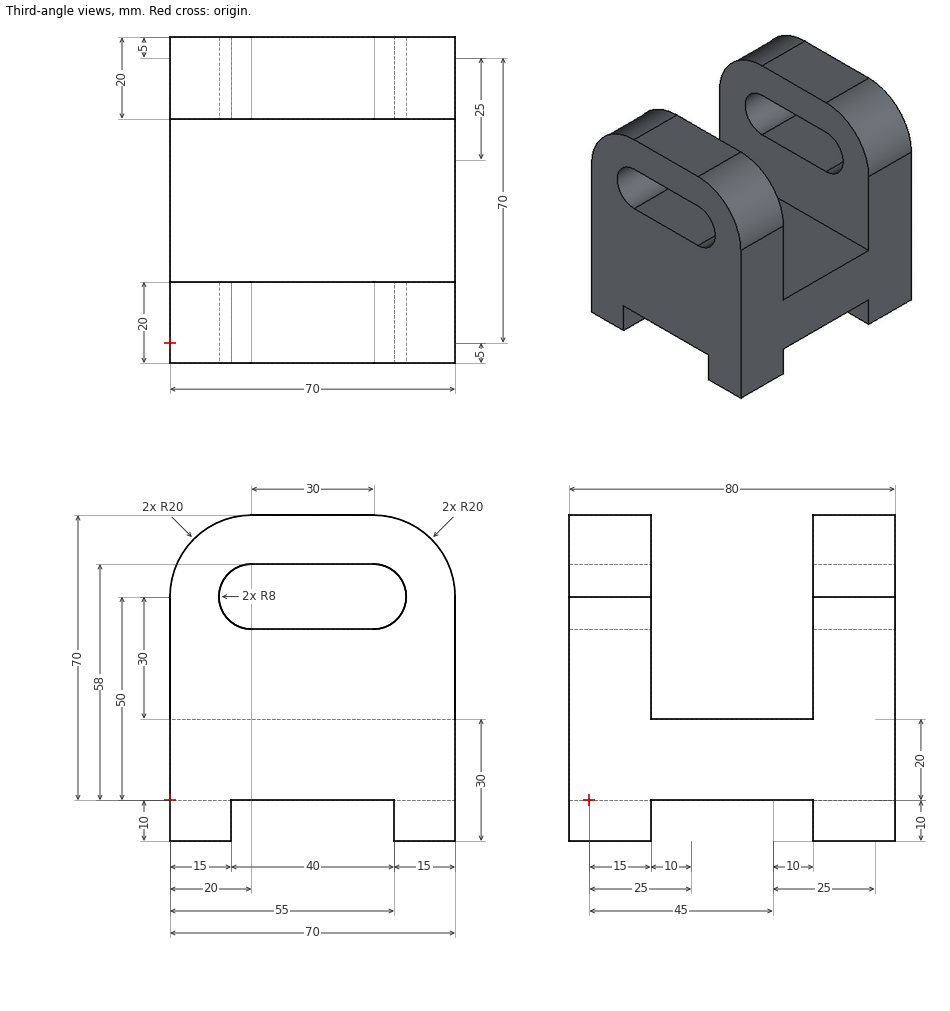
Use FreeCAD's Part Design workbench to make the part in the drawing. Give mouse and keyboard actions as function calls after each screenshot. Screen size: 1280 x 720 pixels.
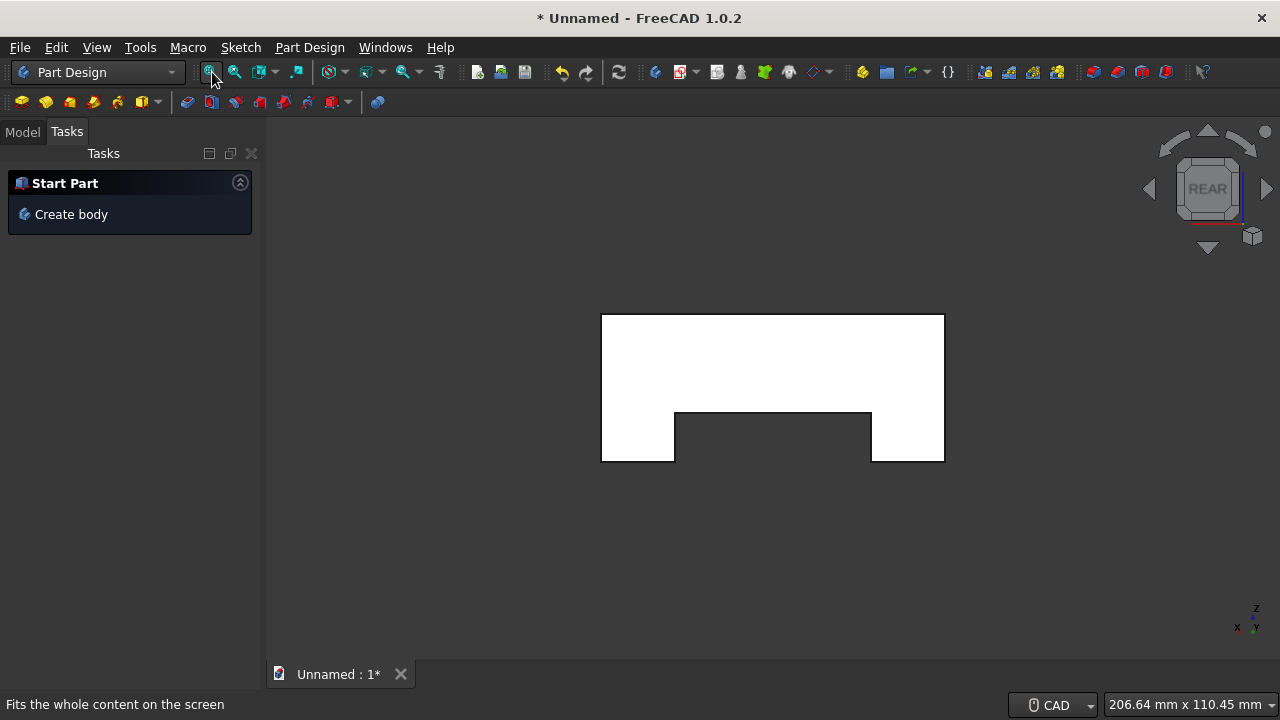
key(0)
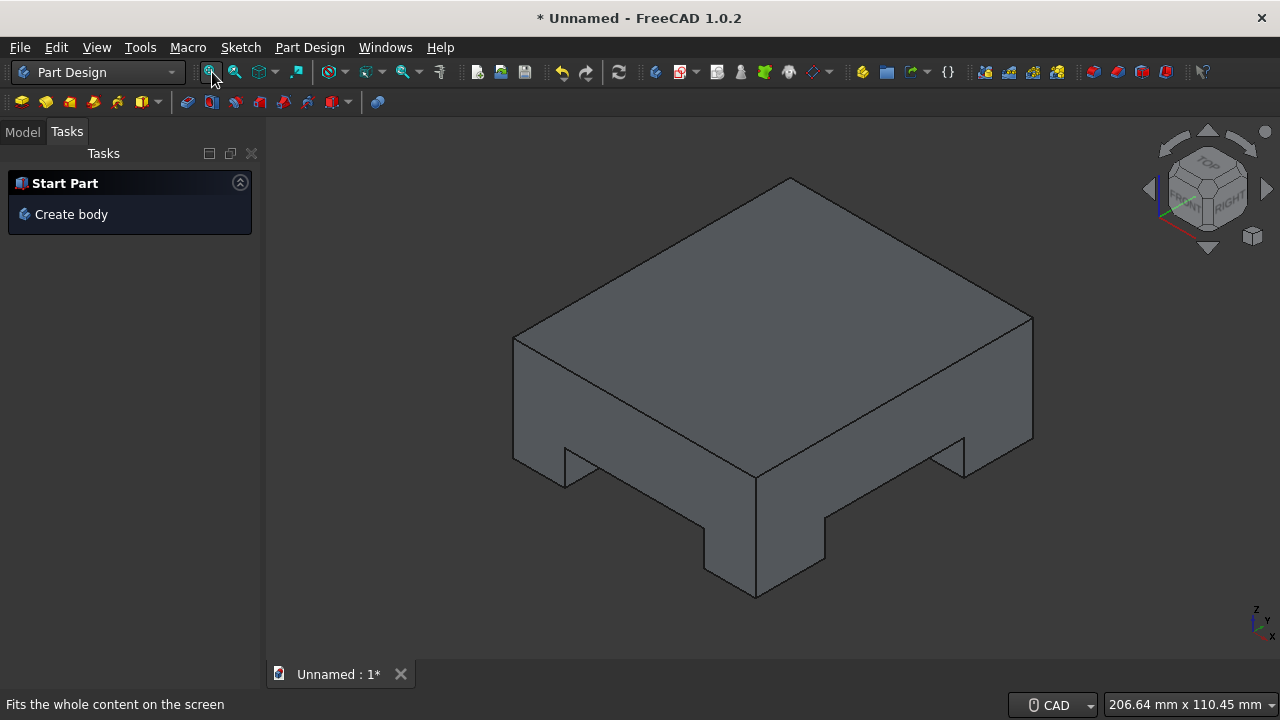
click(704, 490)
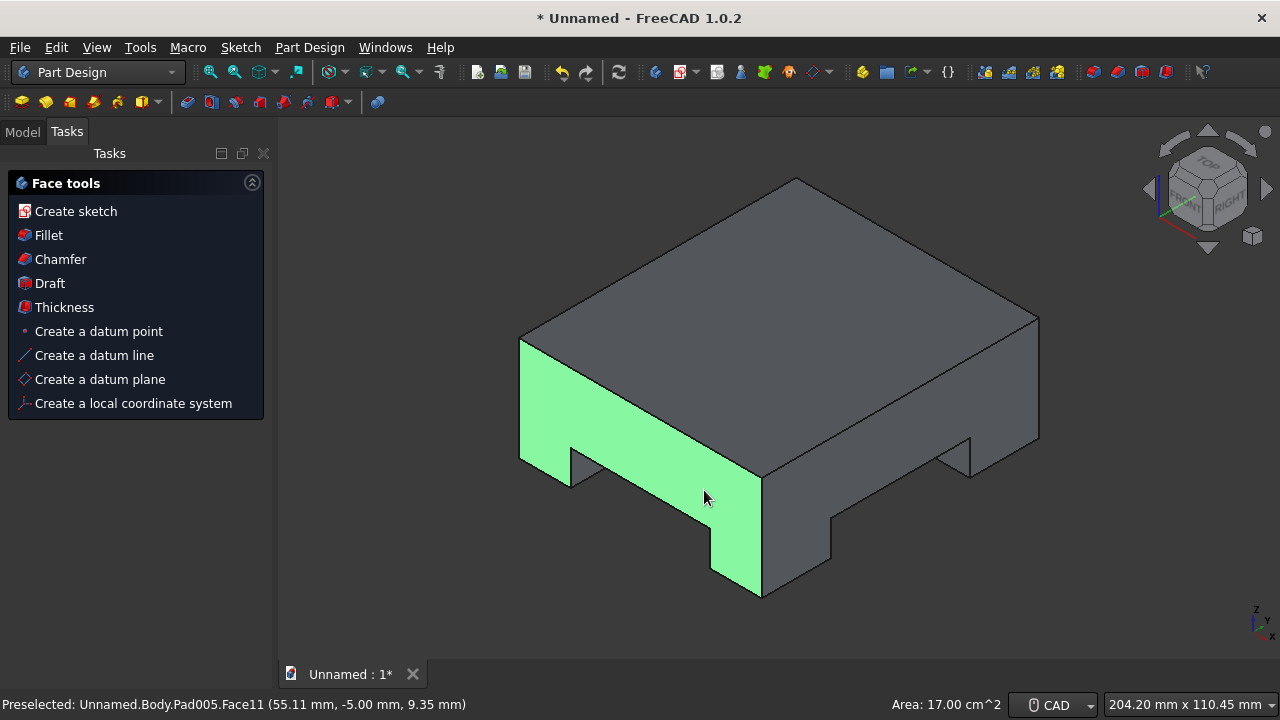
click(680, 72)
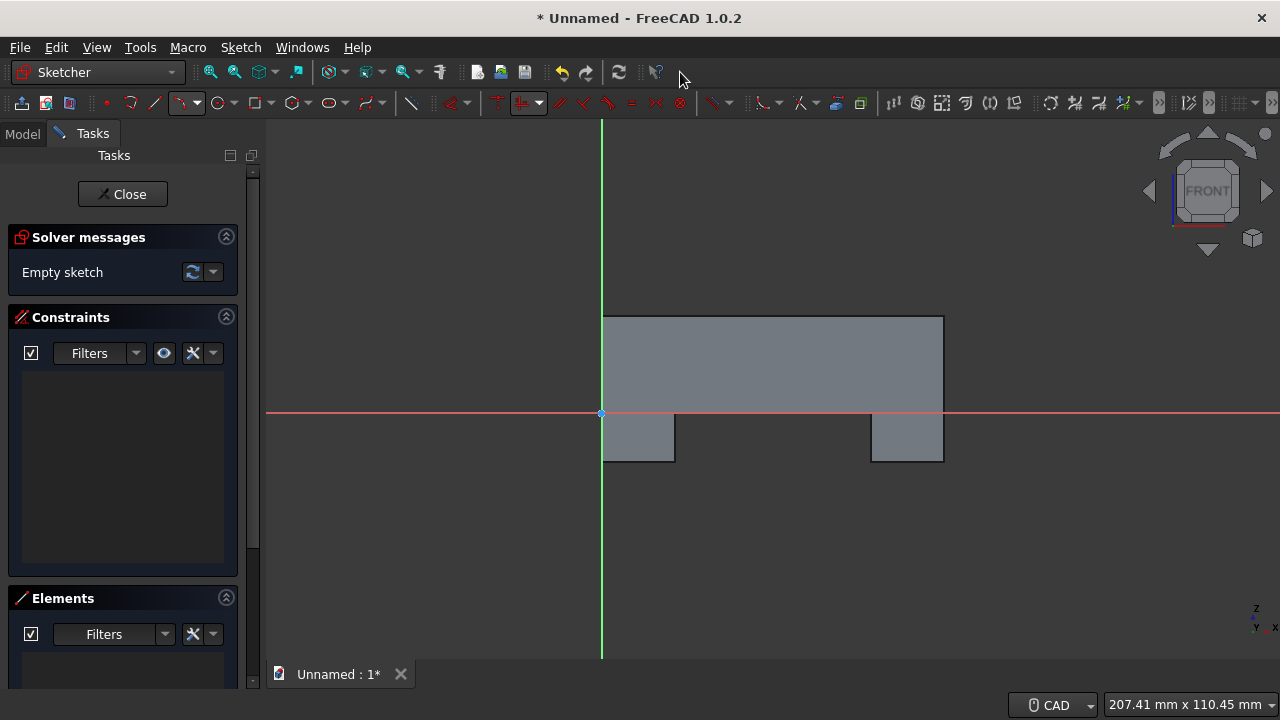
scroll(395, 631, down, 1)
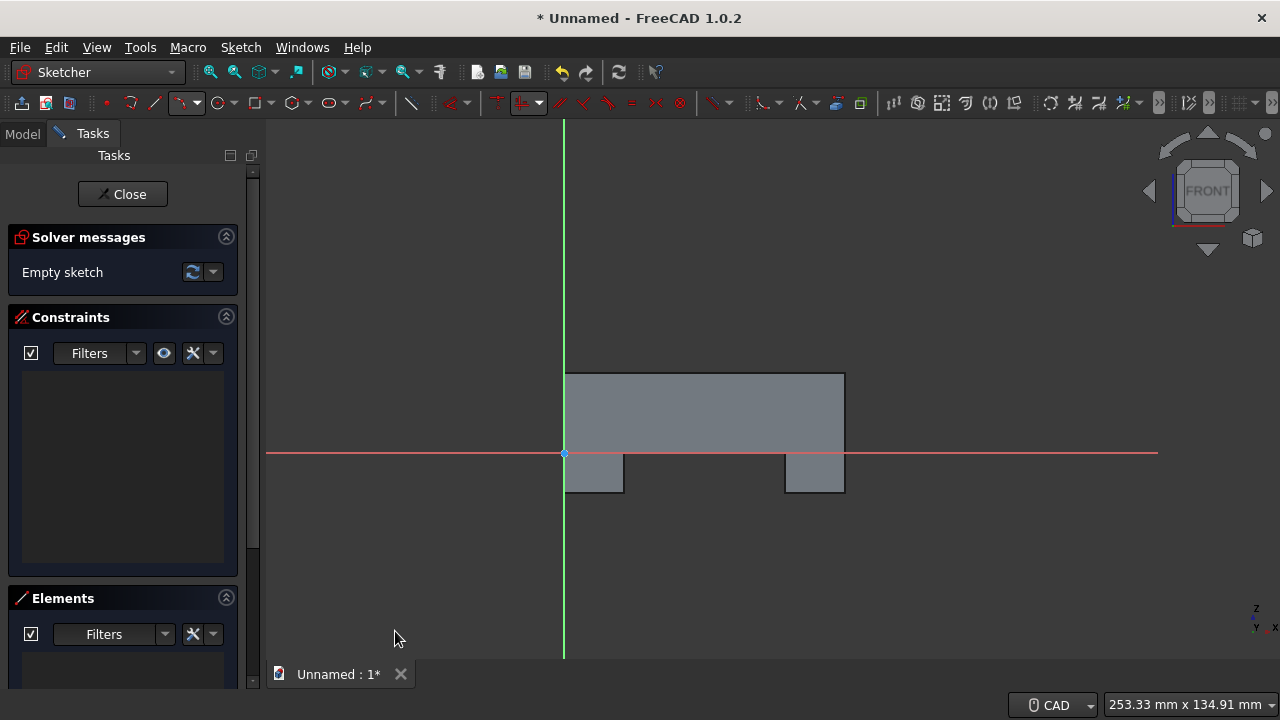
key(g)
key(m)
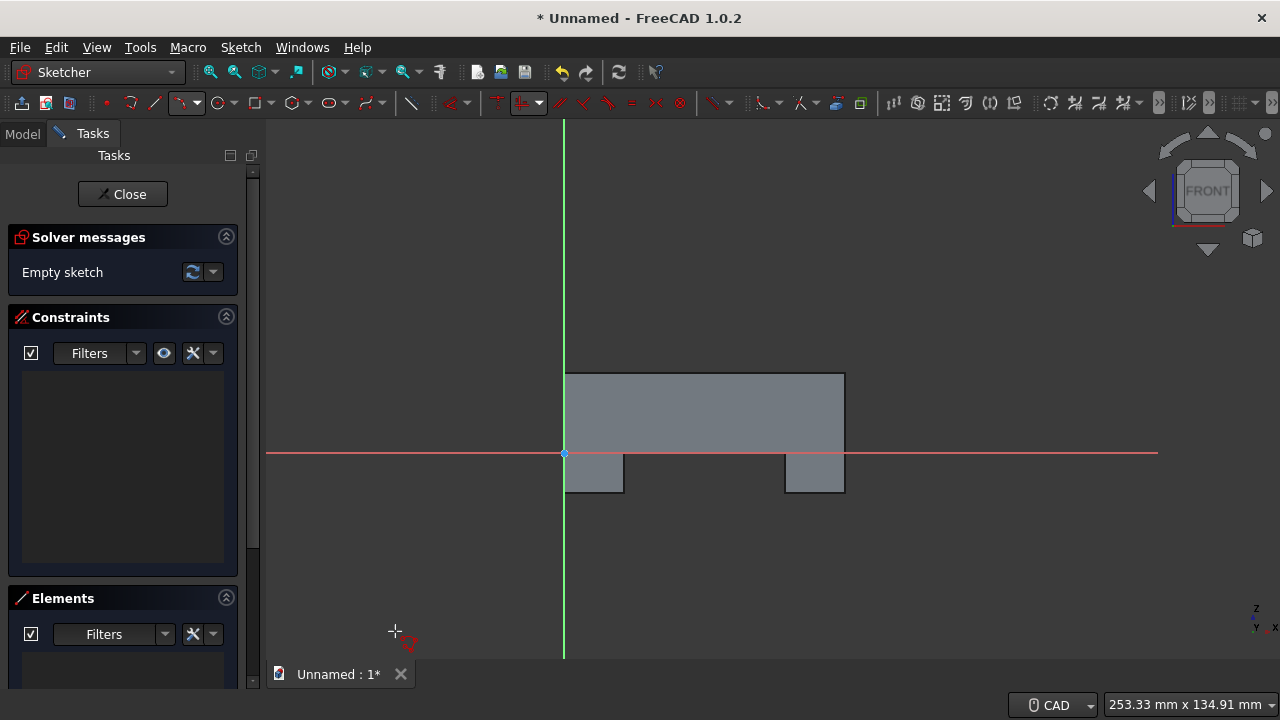
click(564, 253)
click(573, 373)
click(845, 373)
click(845, 253)
right_click(845, 253)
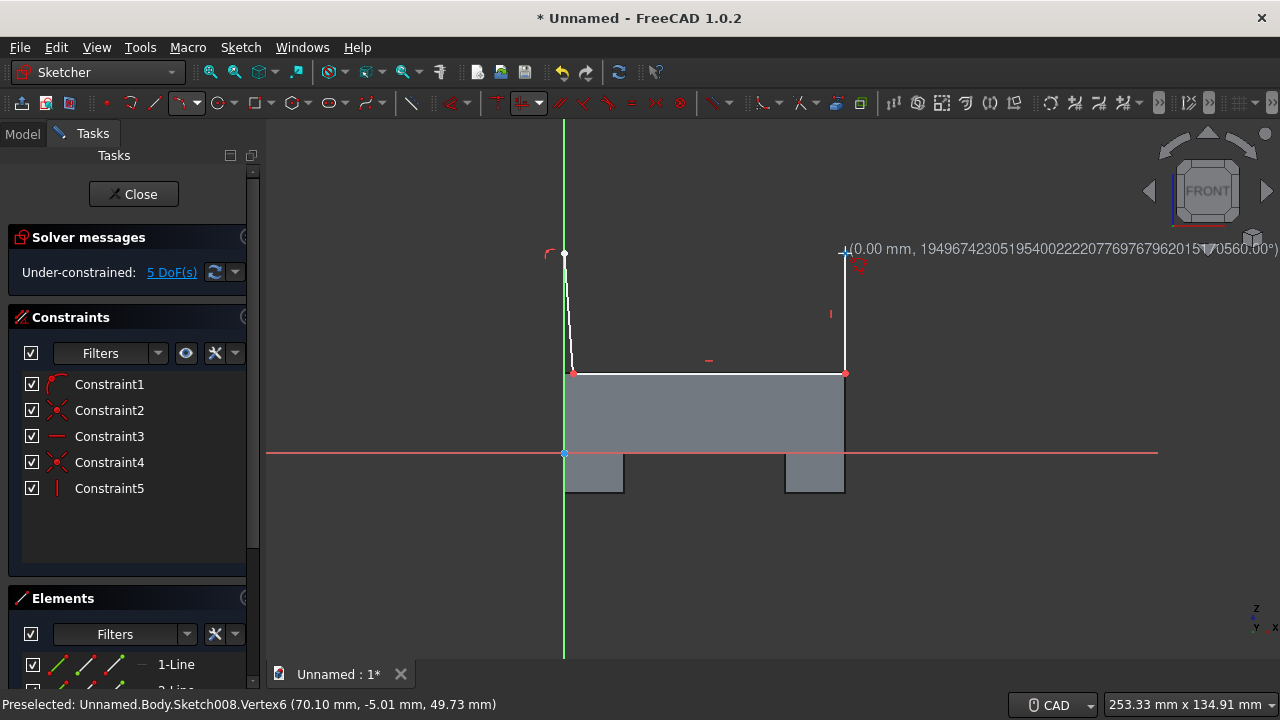
key(g)
key(l)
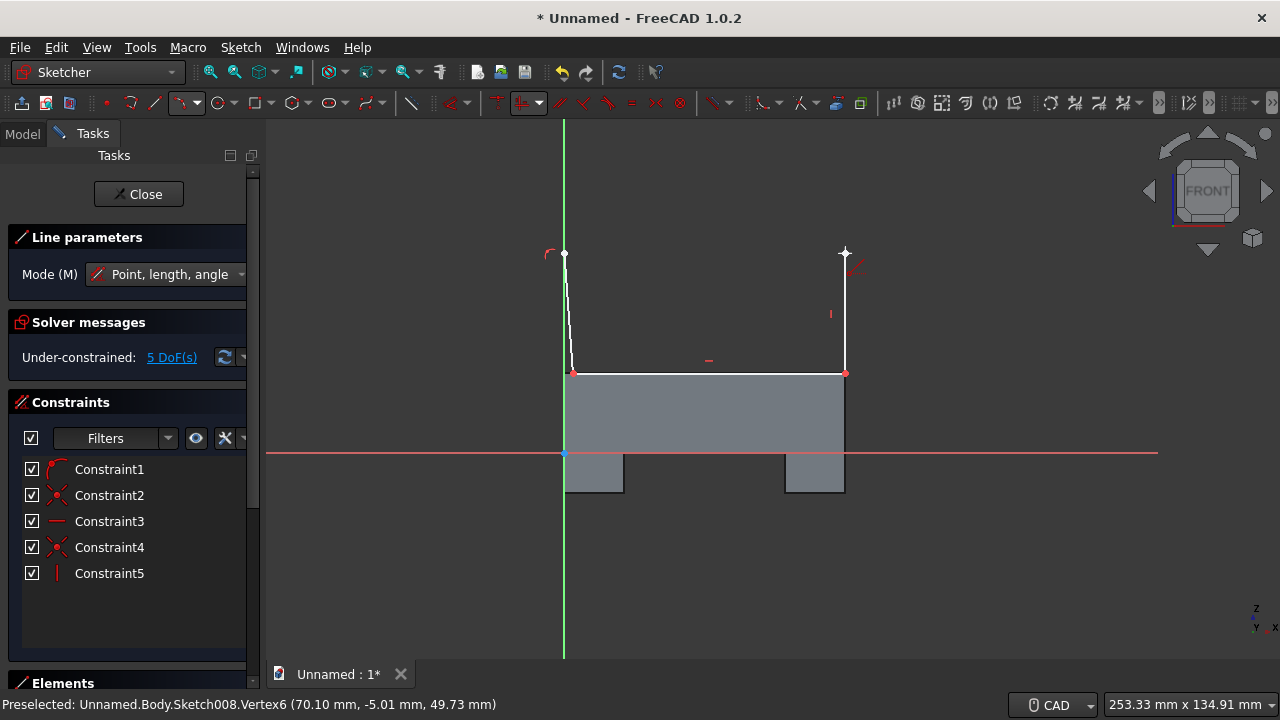
click(765, 173)
click(644, 173)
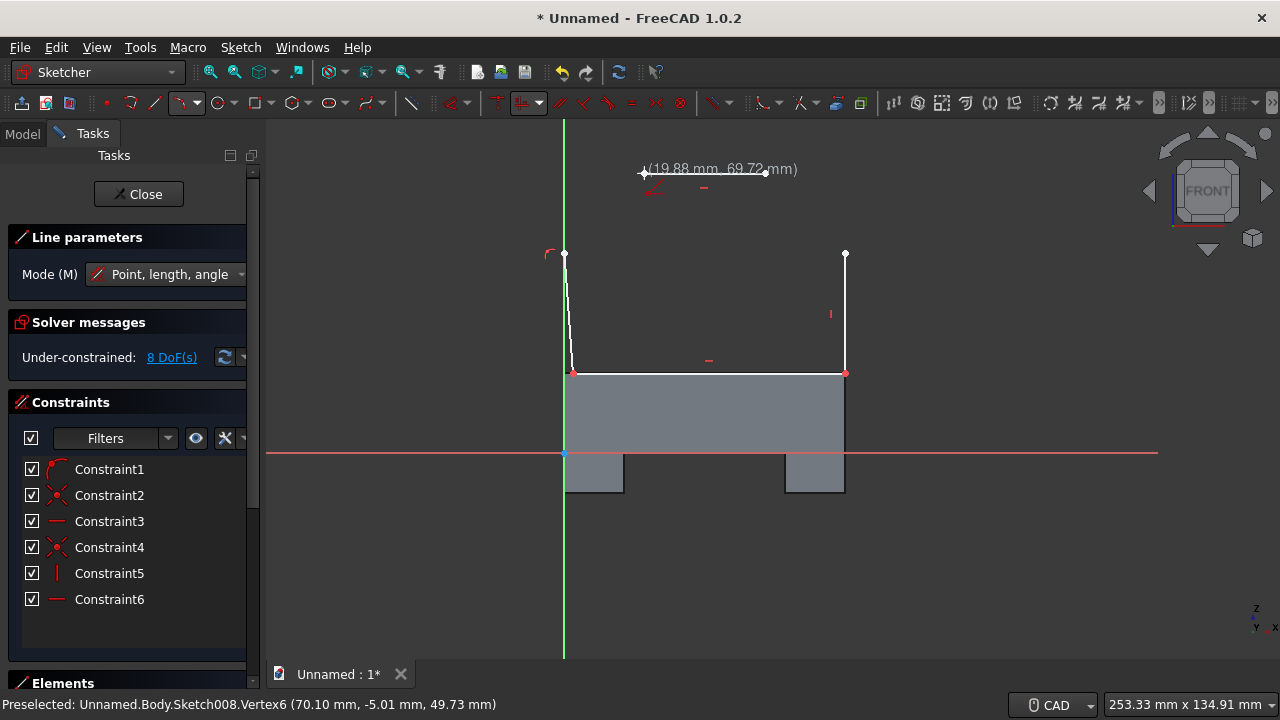
key(g)
key(3)
key(a)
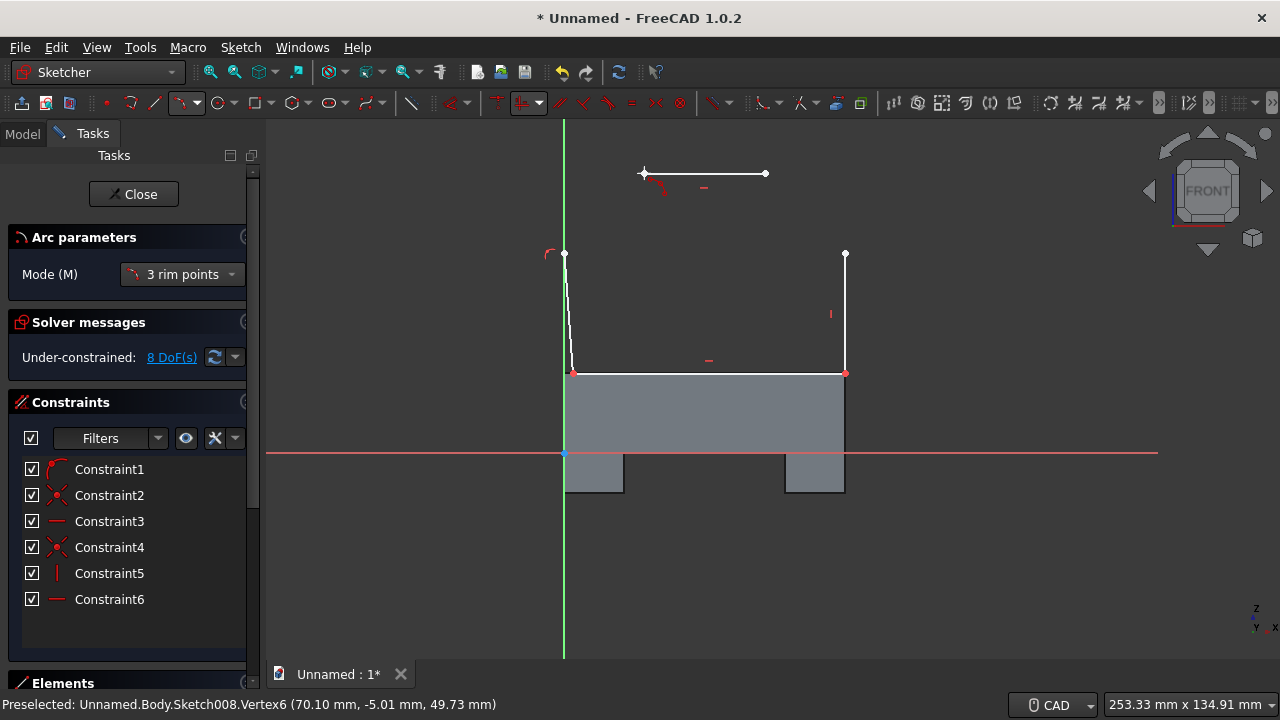
click(845, 254)
click(765, 174)
click(821, 196)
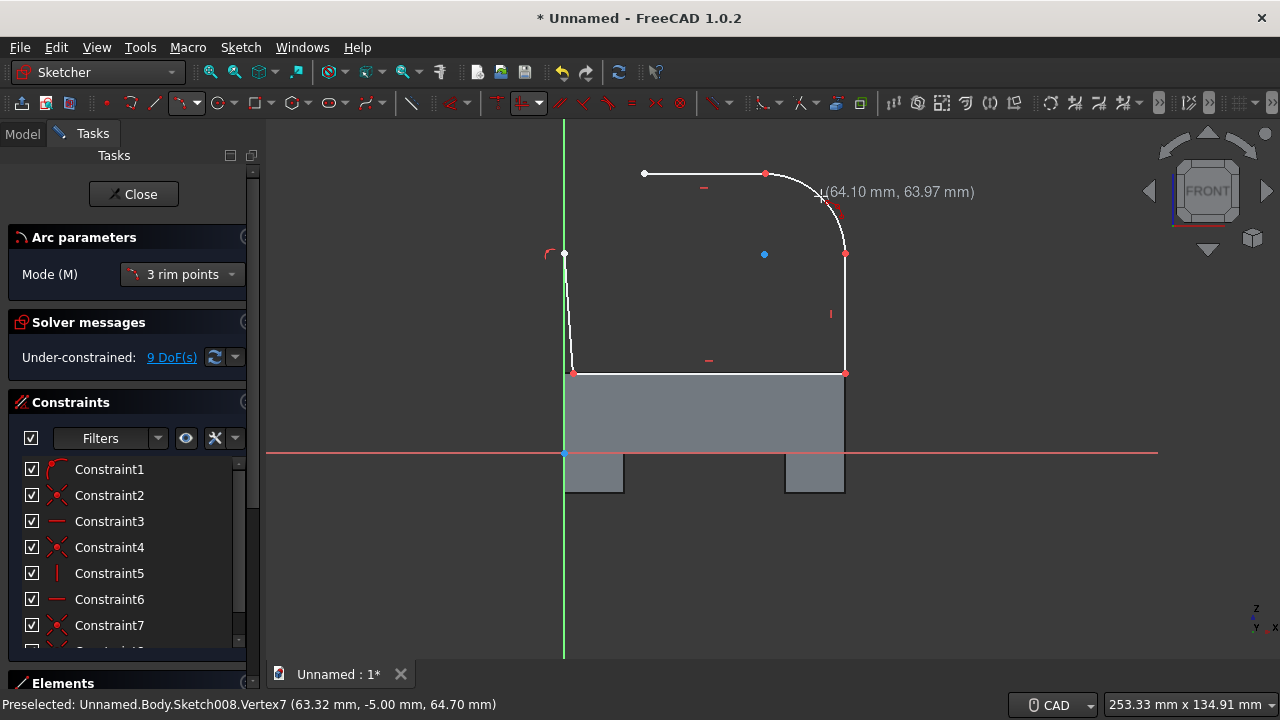
click(644, 174)
click(564, 254)
click(588, 196)
key(Escape)